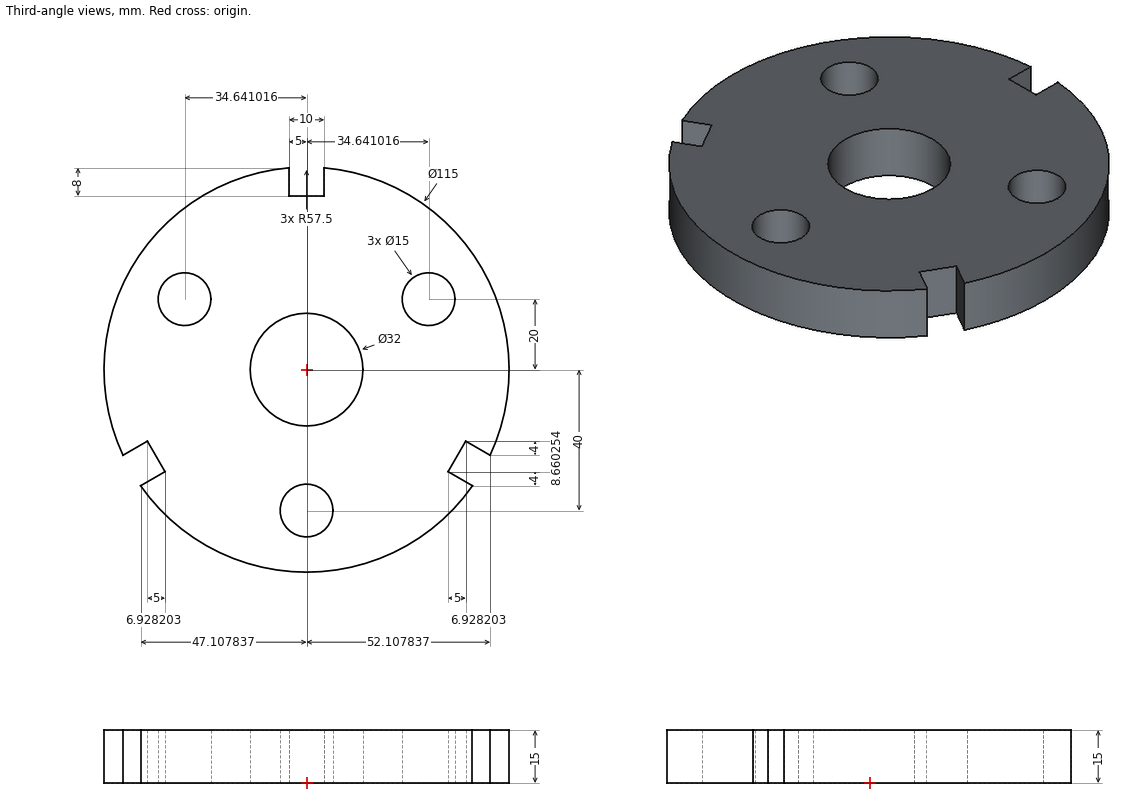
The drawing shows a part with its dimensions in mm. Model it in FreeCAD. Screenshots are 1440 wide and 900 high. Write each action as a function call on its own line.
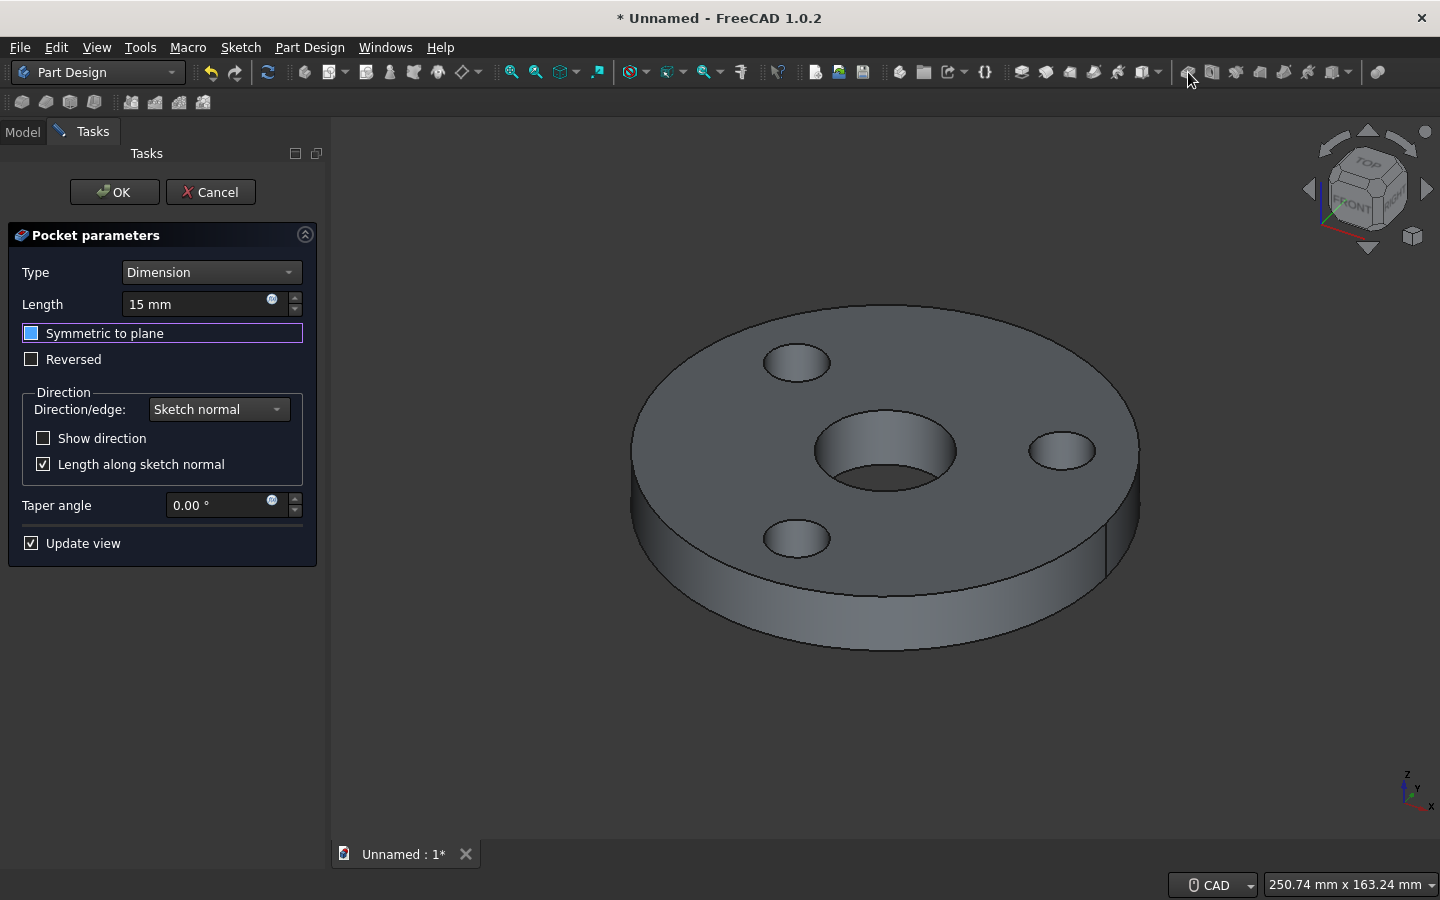
click(115, 192)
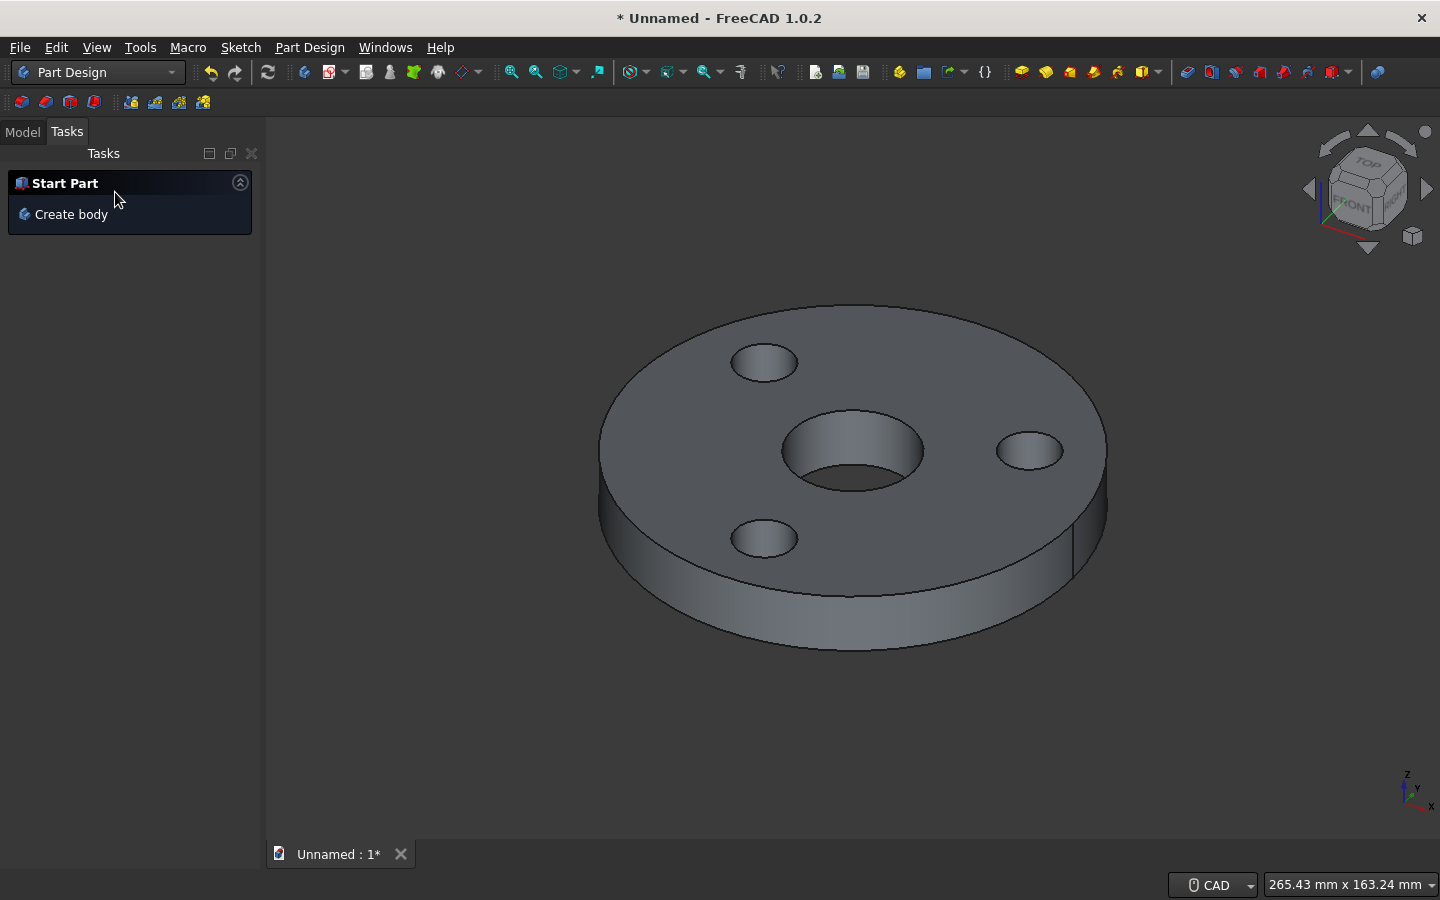
key(5)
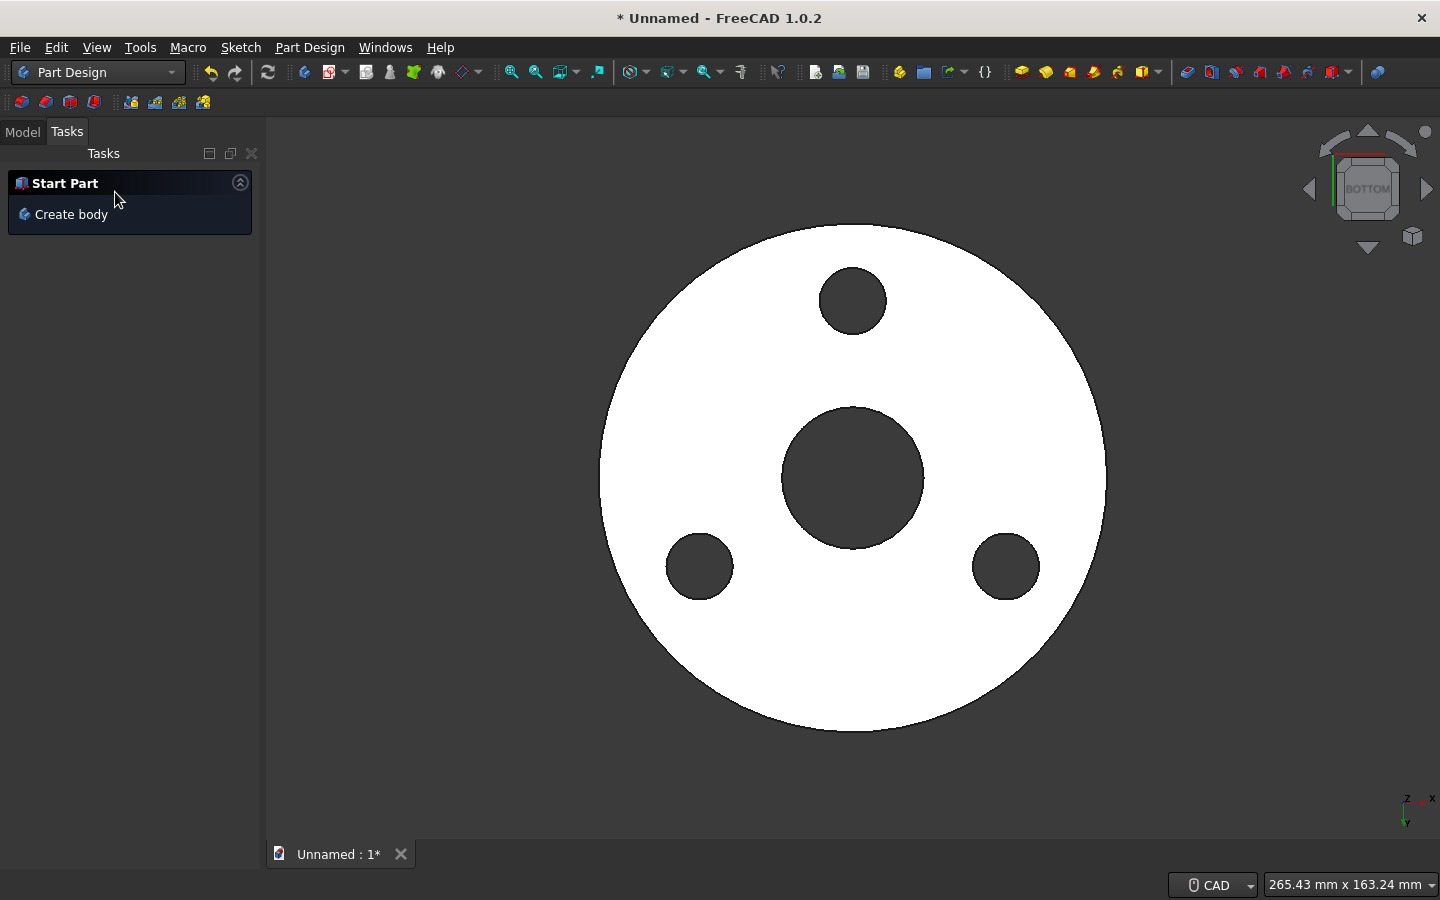
click(998, 404)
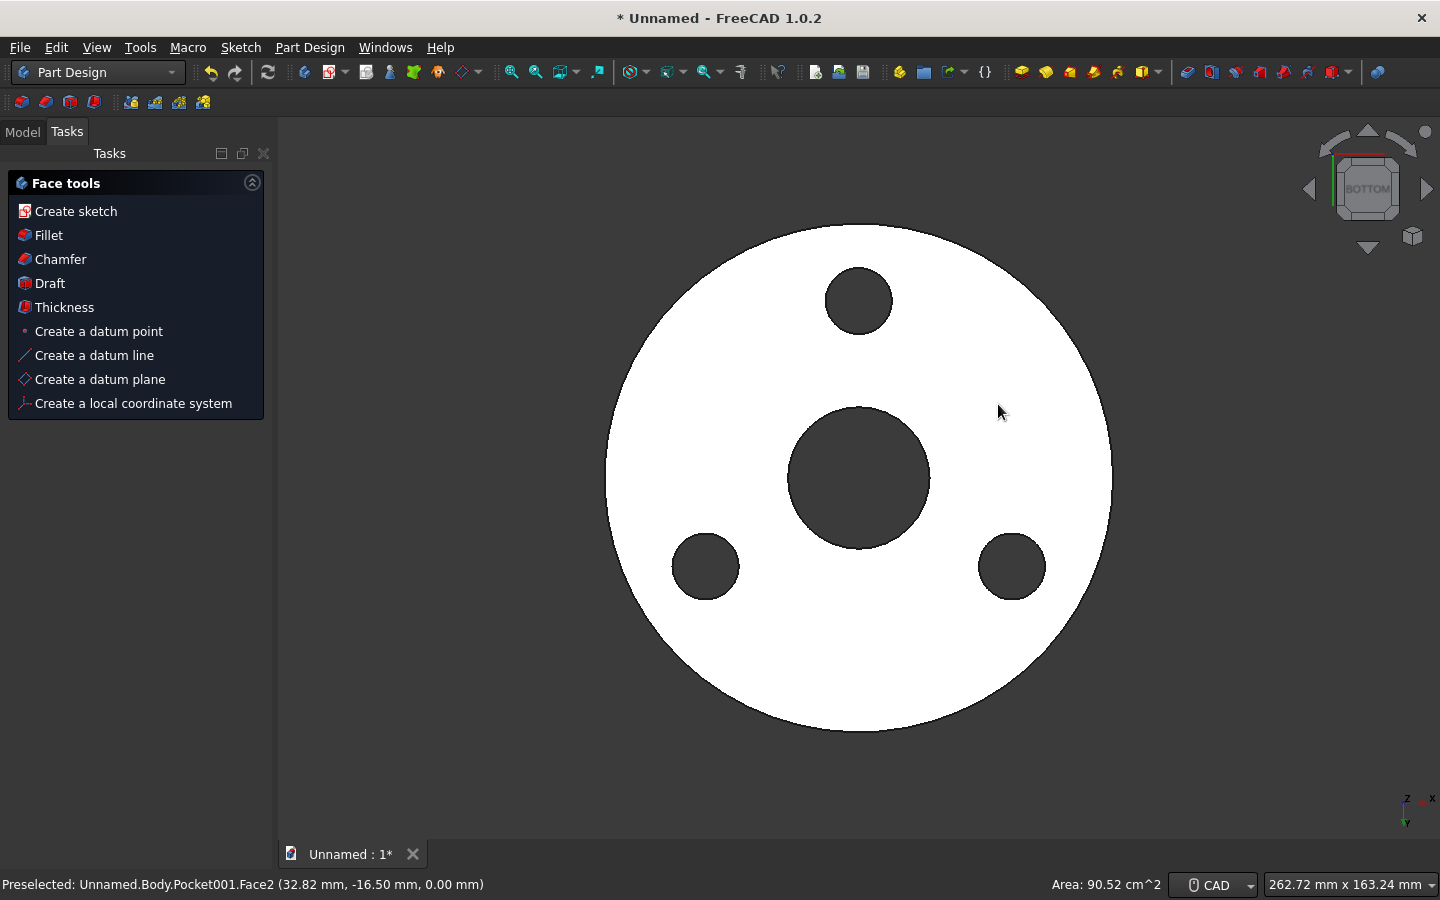
click(330, 72)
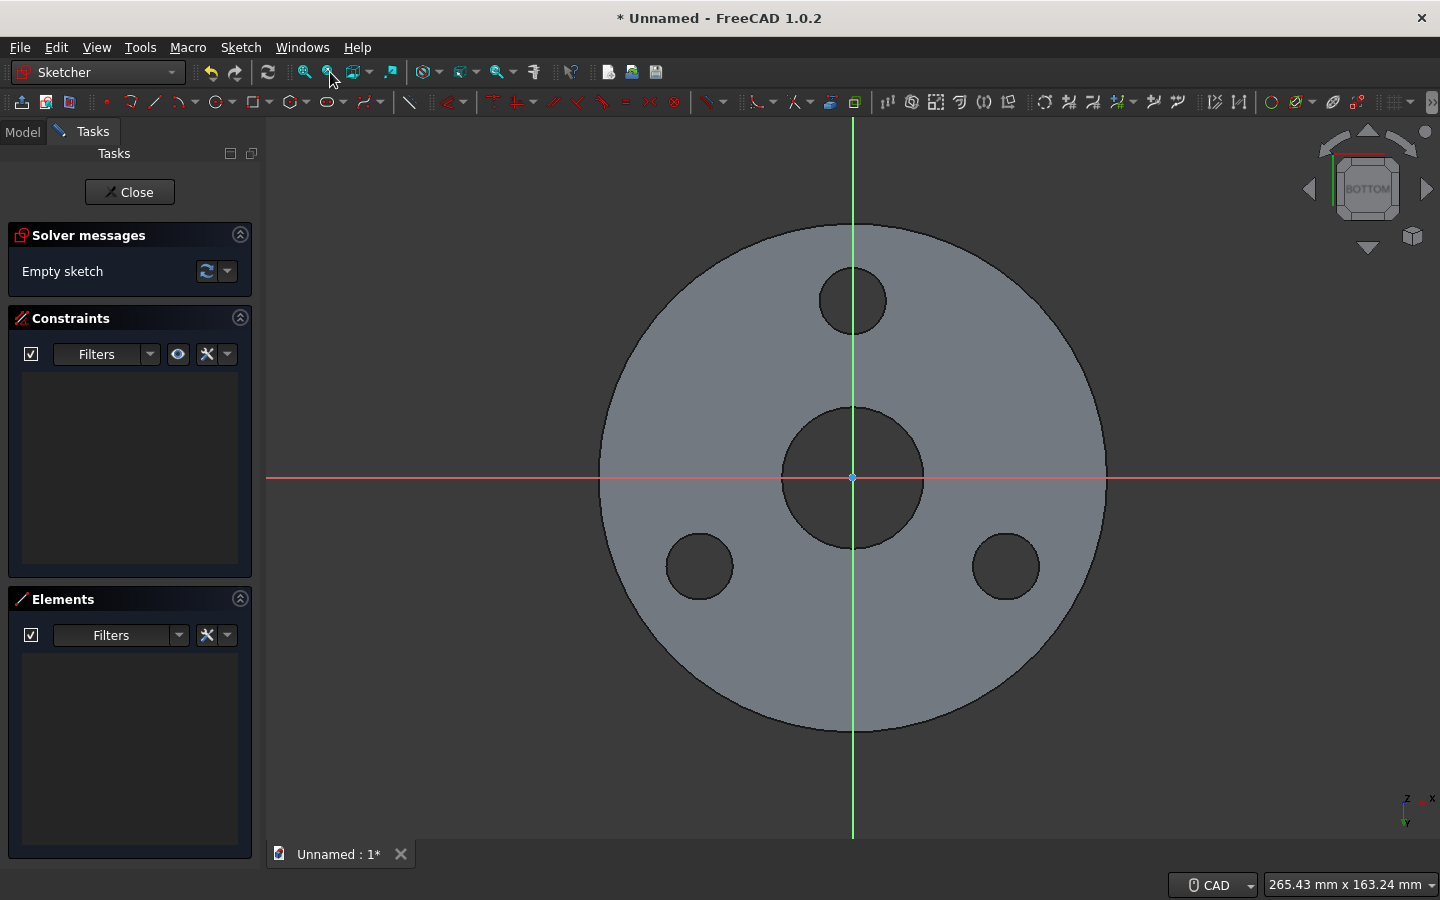
click(132, 102)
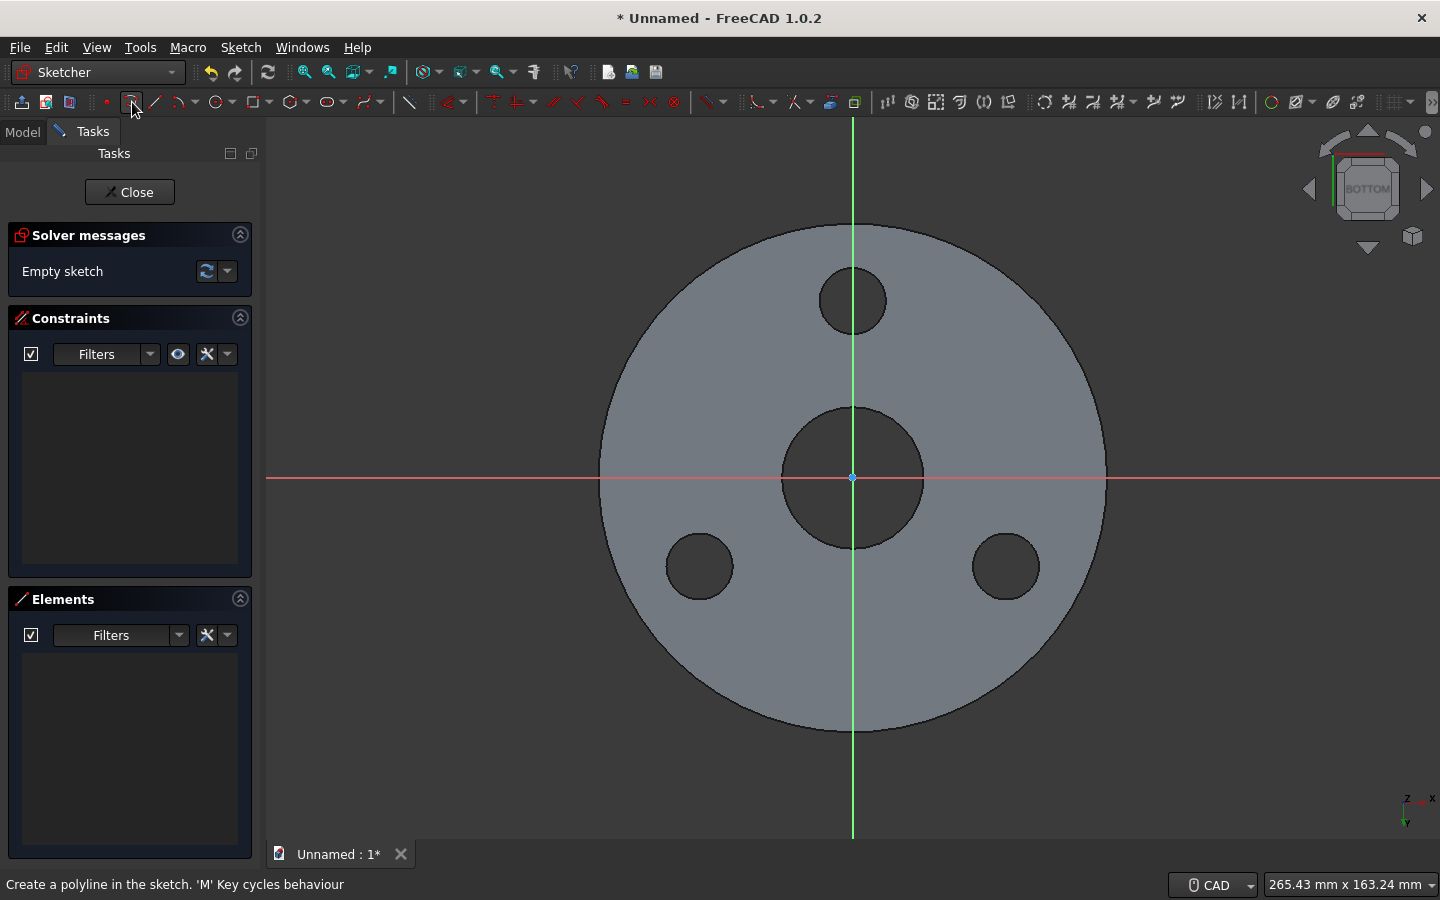
click(831, 731)
click(831, 696)
click(875, 696)
click(875, 731)
right_click(875, 731)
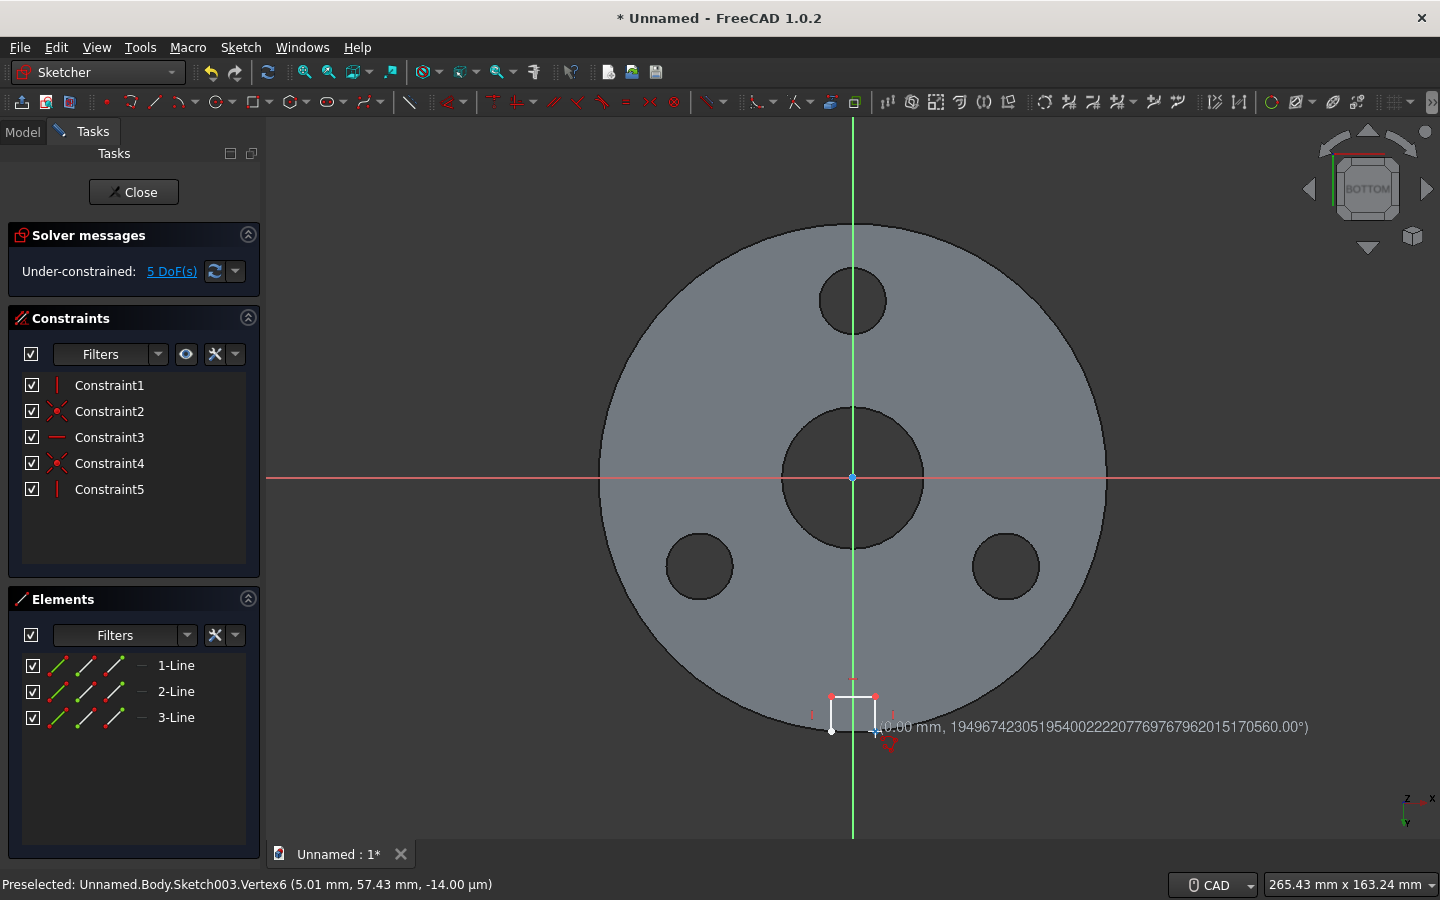
key(g)
key(3)
key(a)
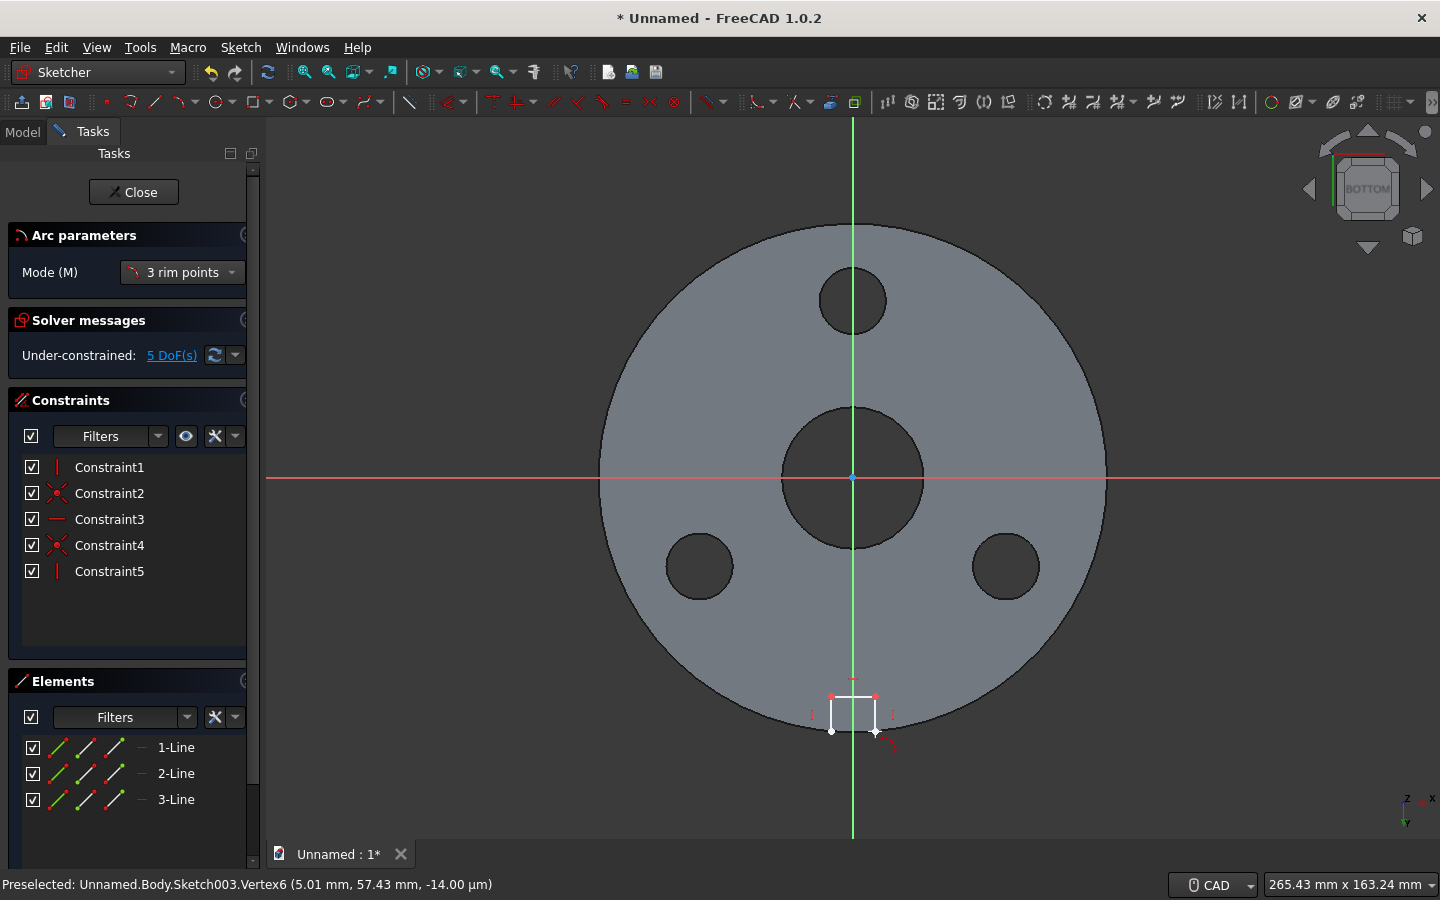
click(875, 732)
click(831, 732)